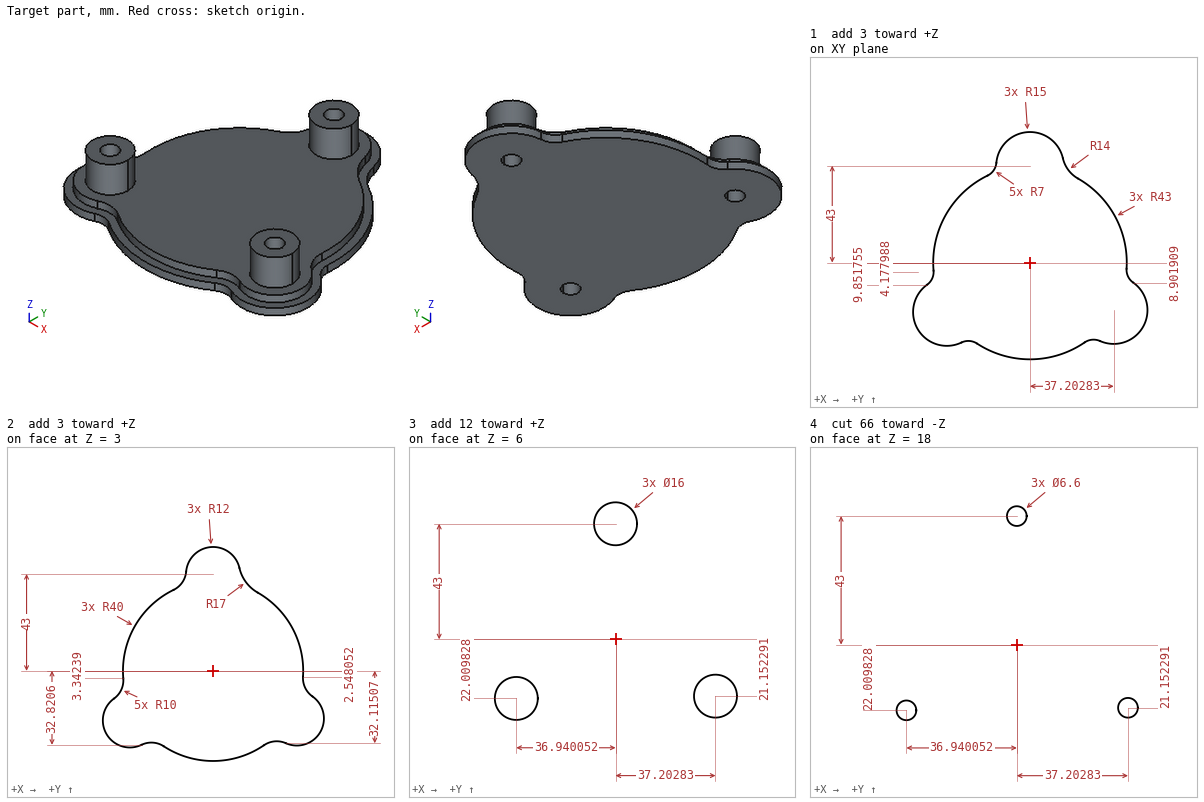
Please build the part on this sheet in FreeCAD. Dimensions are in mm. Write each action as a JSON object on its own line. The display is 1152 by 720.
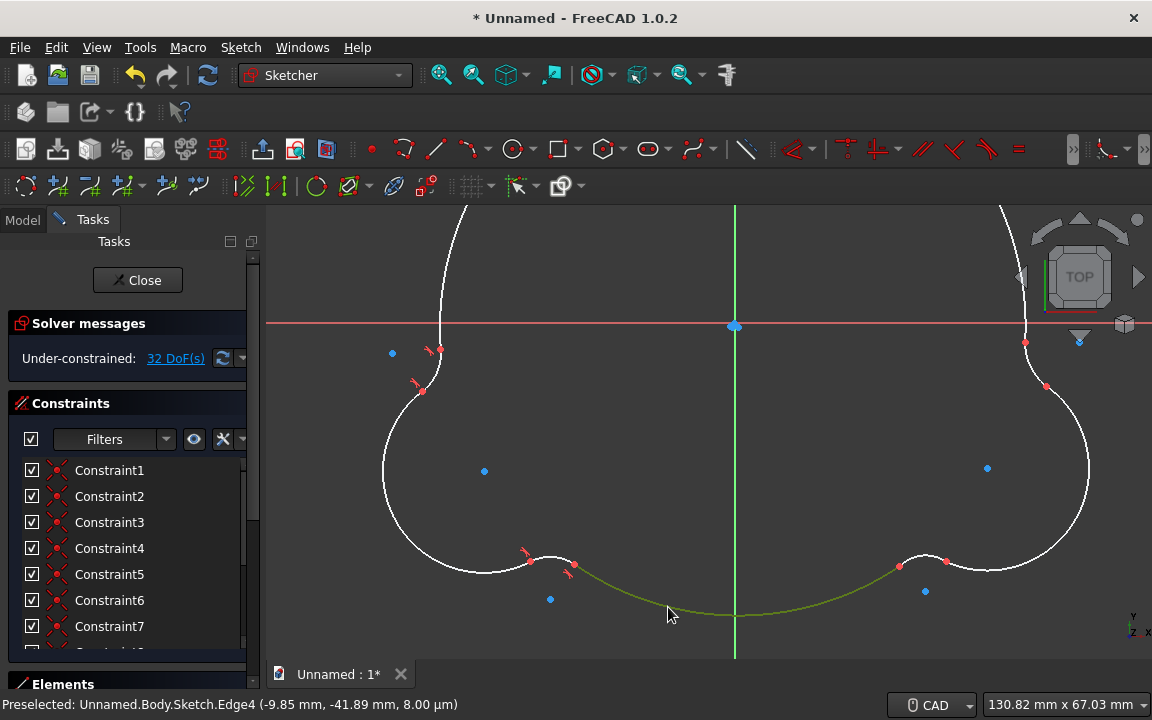
{"action": "left_click", "coordinate": [932, 556]}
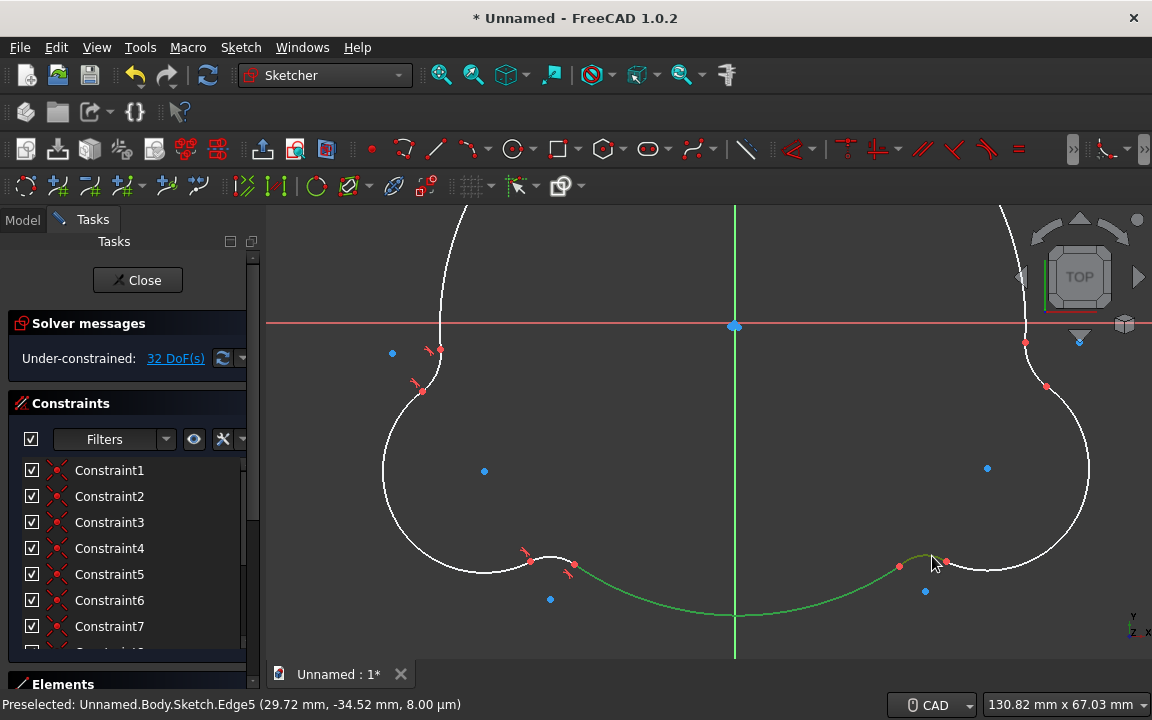
{"action": "left_click", "coordinate": [988, 150]}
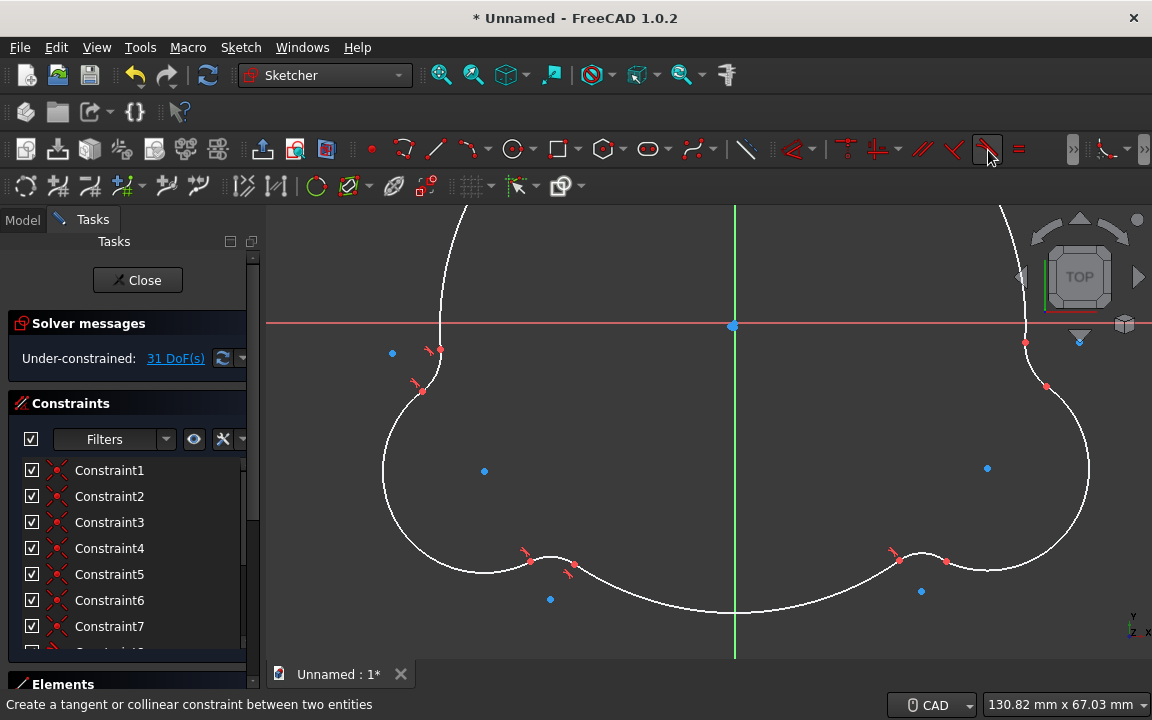
{"action": "left_click", "coordinate": [933, 555]}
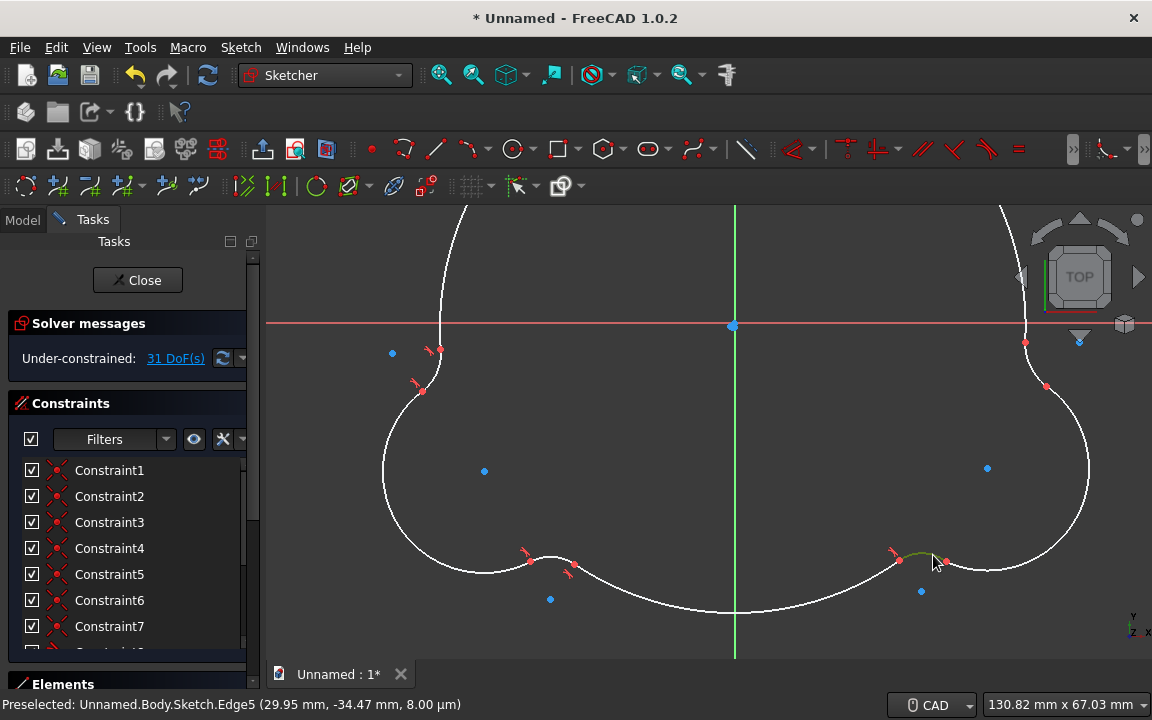
{"action": "scroll", "coordinate": [562, 562], "scroll_direction": "down", "scroll_amount": 4}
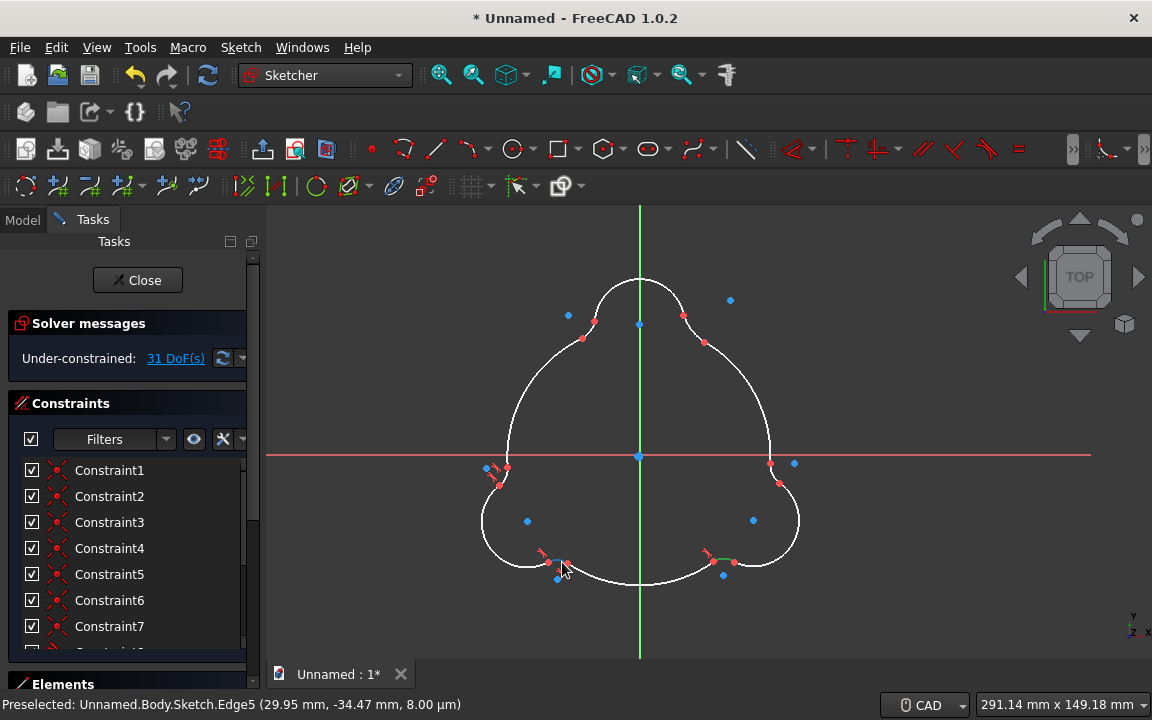
{"action": "left_click", "coordinate": [774, 561]}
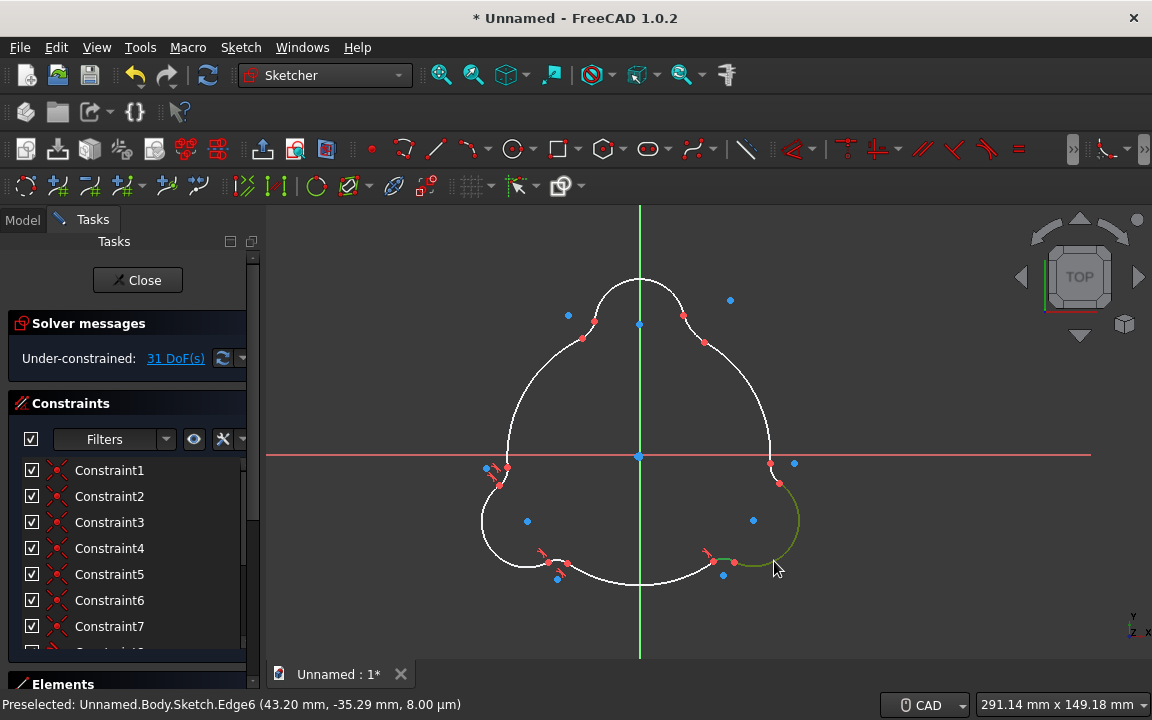
{"action": "left_click", "coordinate": [988, 150]}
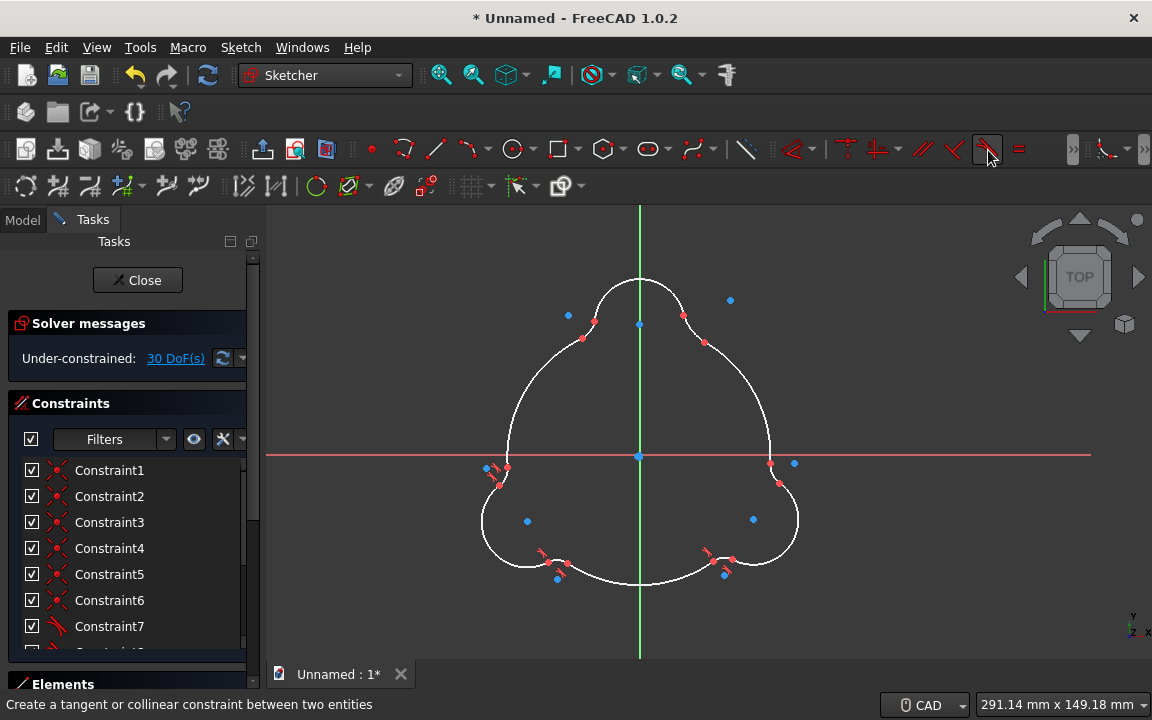
{"action": "left_click", "coordinate": [772, 561]}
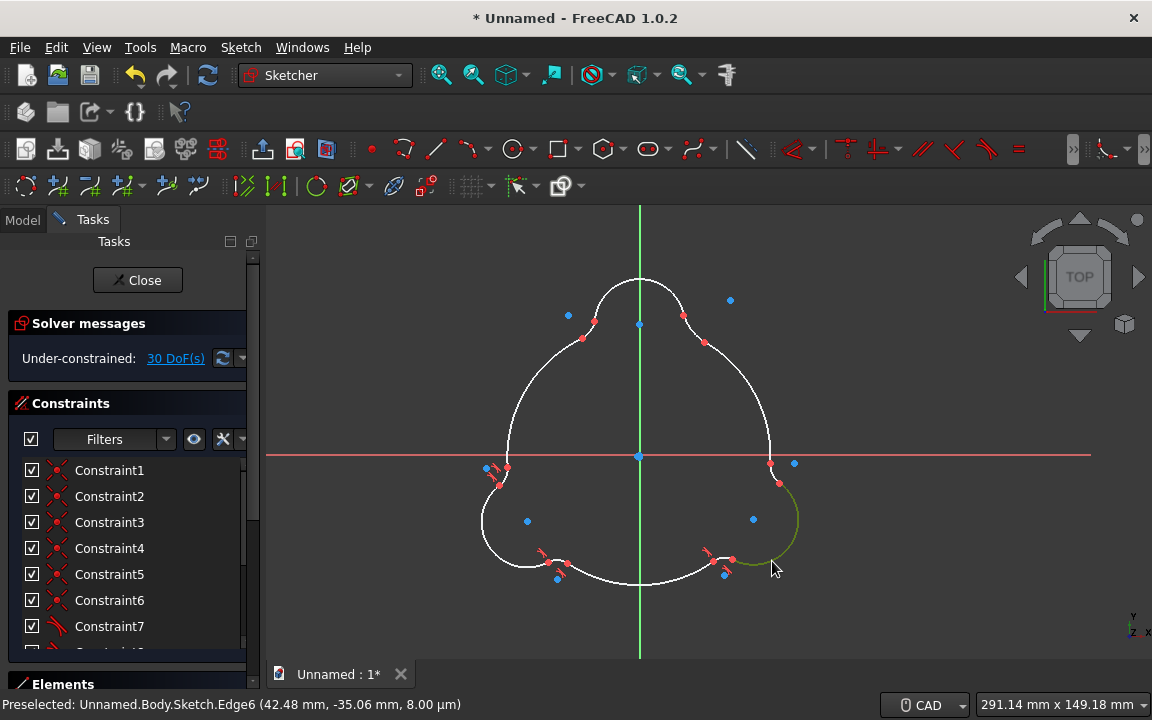
{"action": "scroll", "coordinate": [773, 475], "scroll_direction": "up", "scroll_amount": 2}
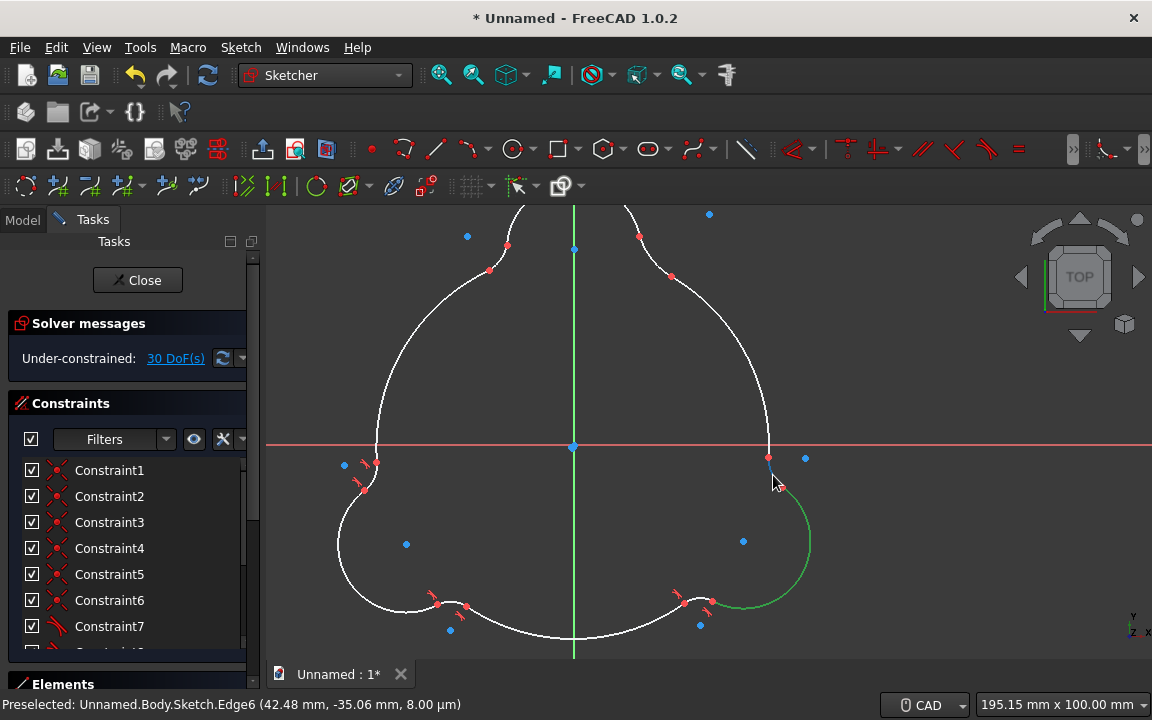
{"action": "left_click", "coordinate": [772, 474]}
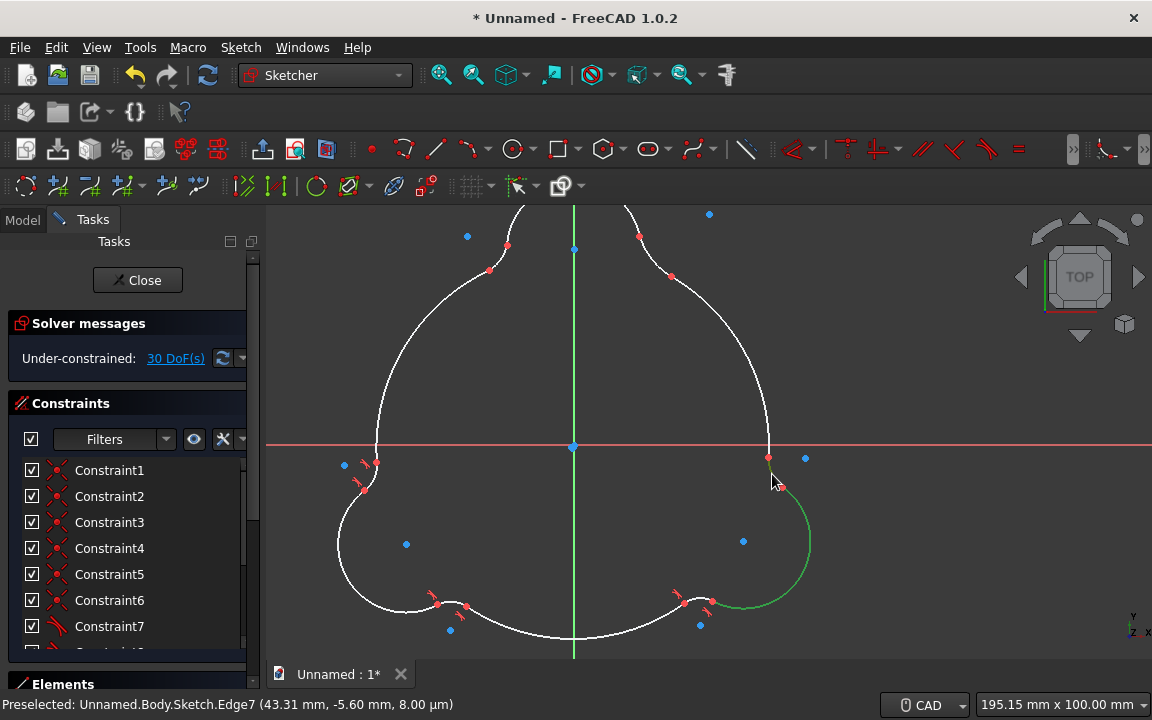
{"action": "left_click", "coordinate": [988, 150]}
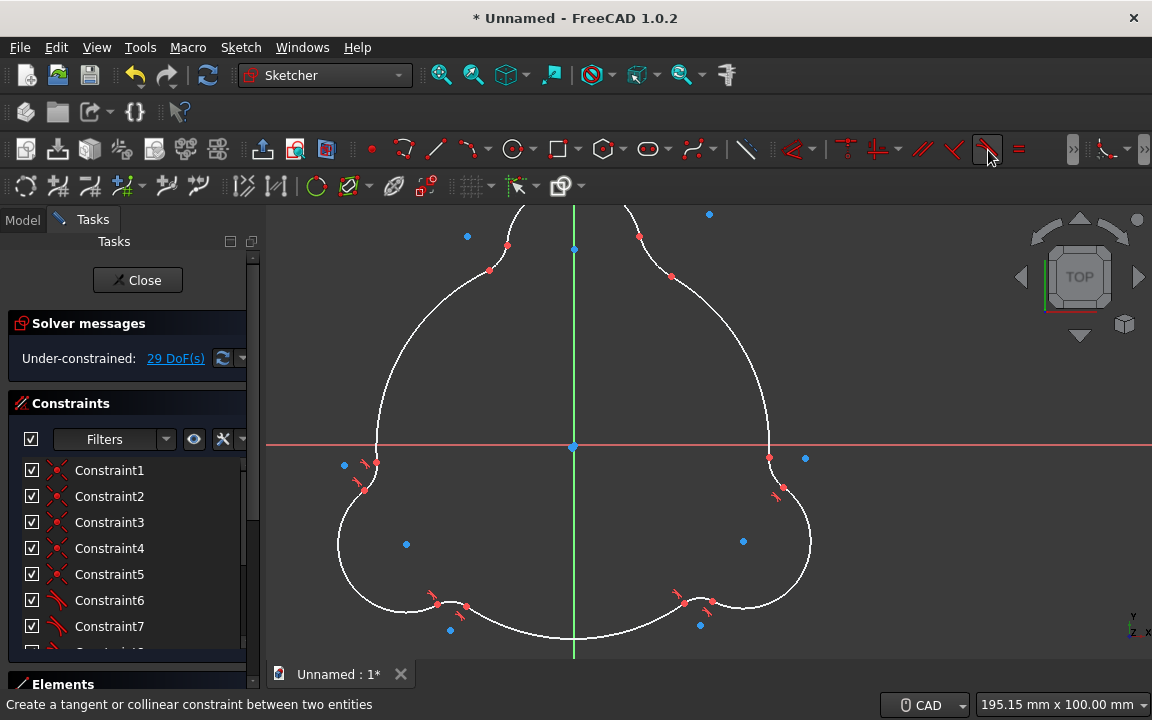
{"action": "scroll", "coordinate": [770, 468], "scroll_direction": "up", "scroll_amount": 2}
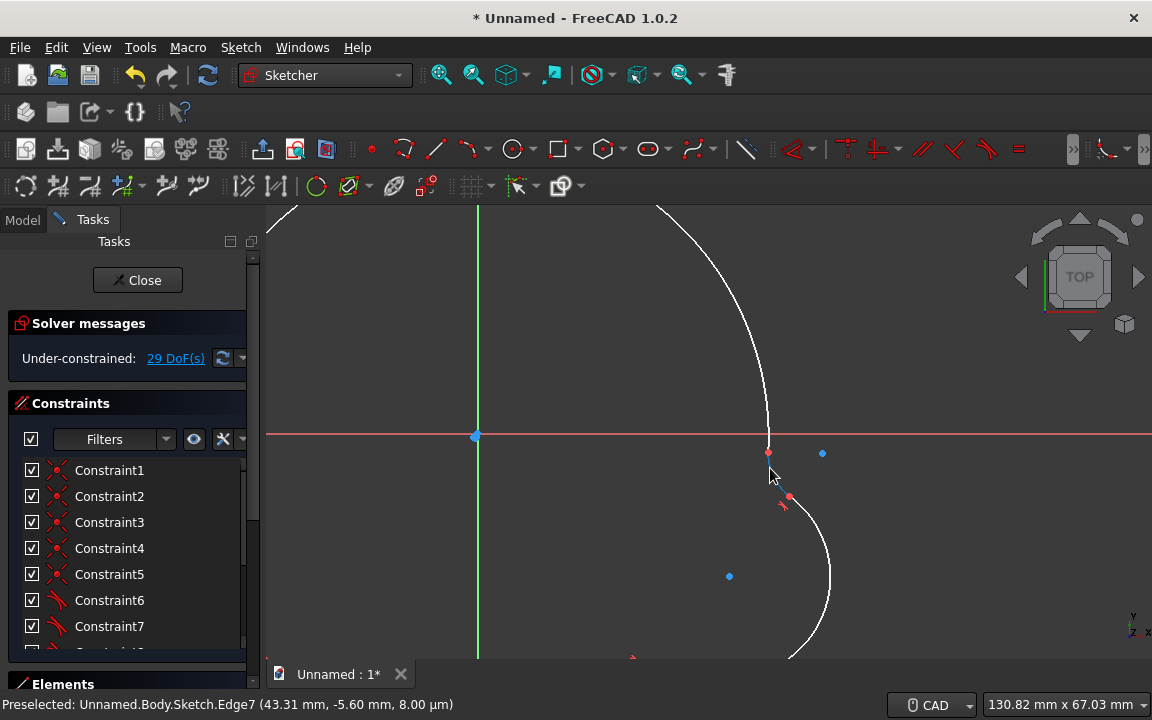
{"action": "left_click", "coordinate": [770, 468]}